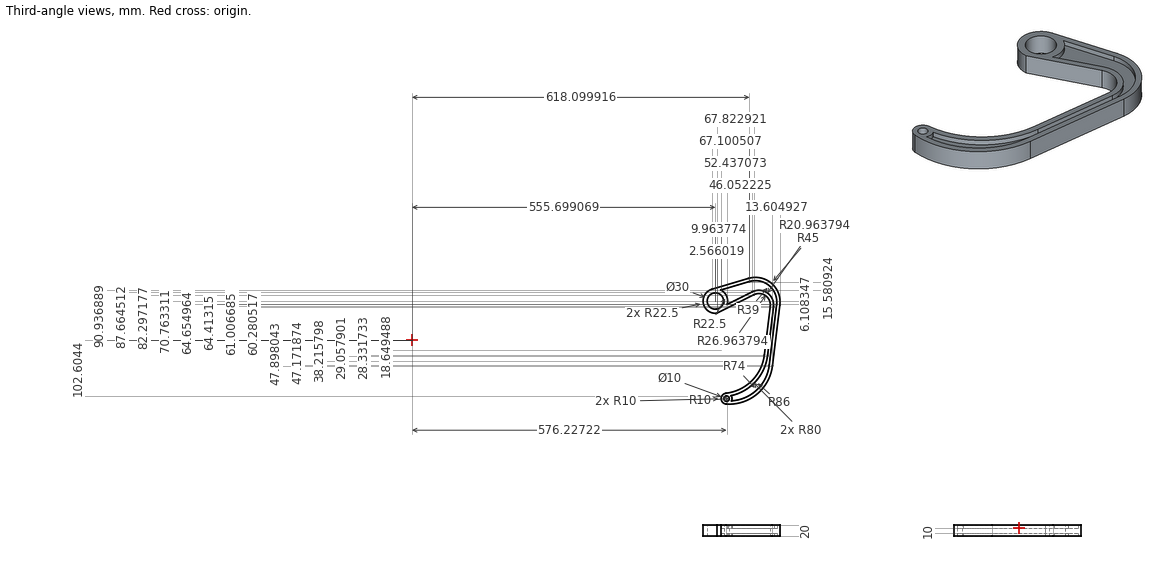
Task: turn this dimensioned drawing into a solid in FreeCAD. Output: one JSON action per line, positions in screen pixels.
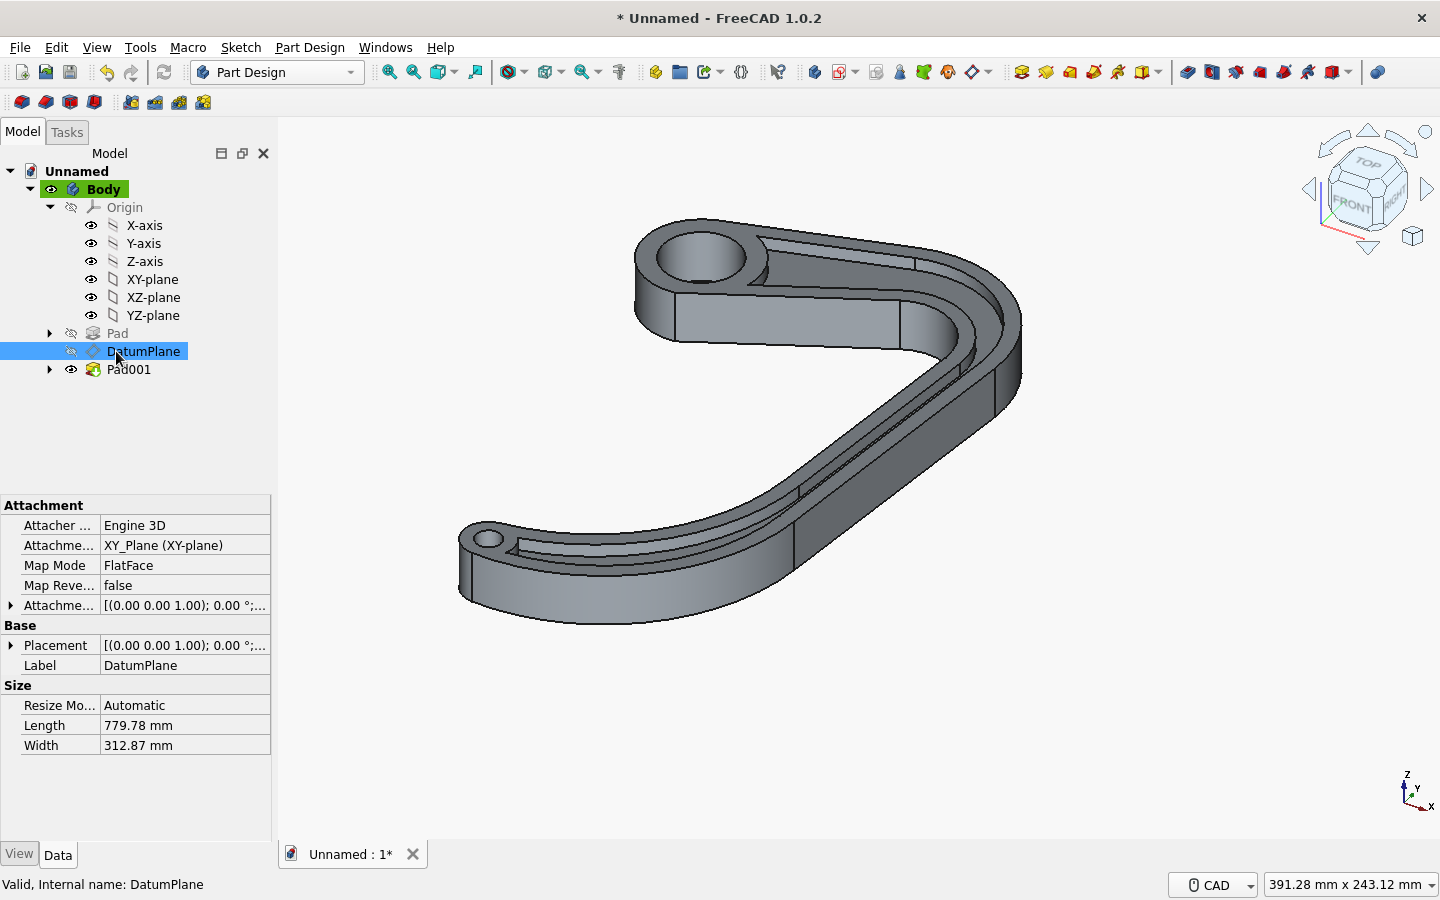
{"action": "key", "text": "0"}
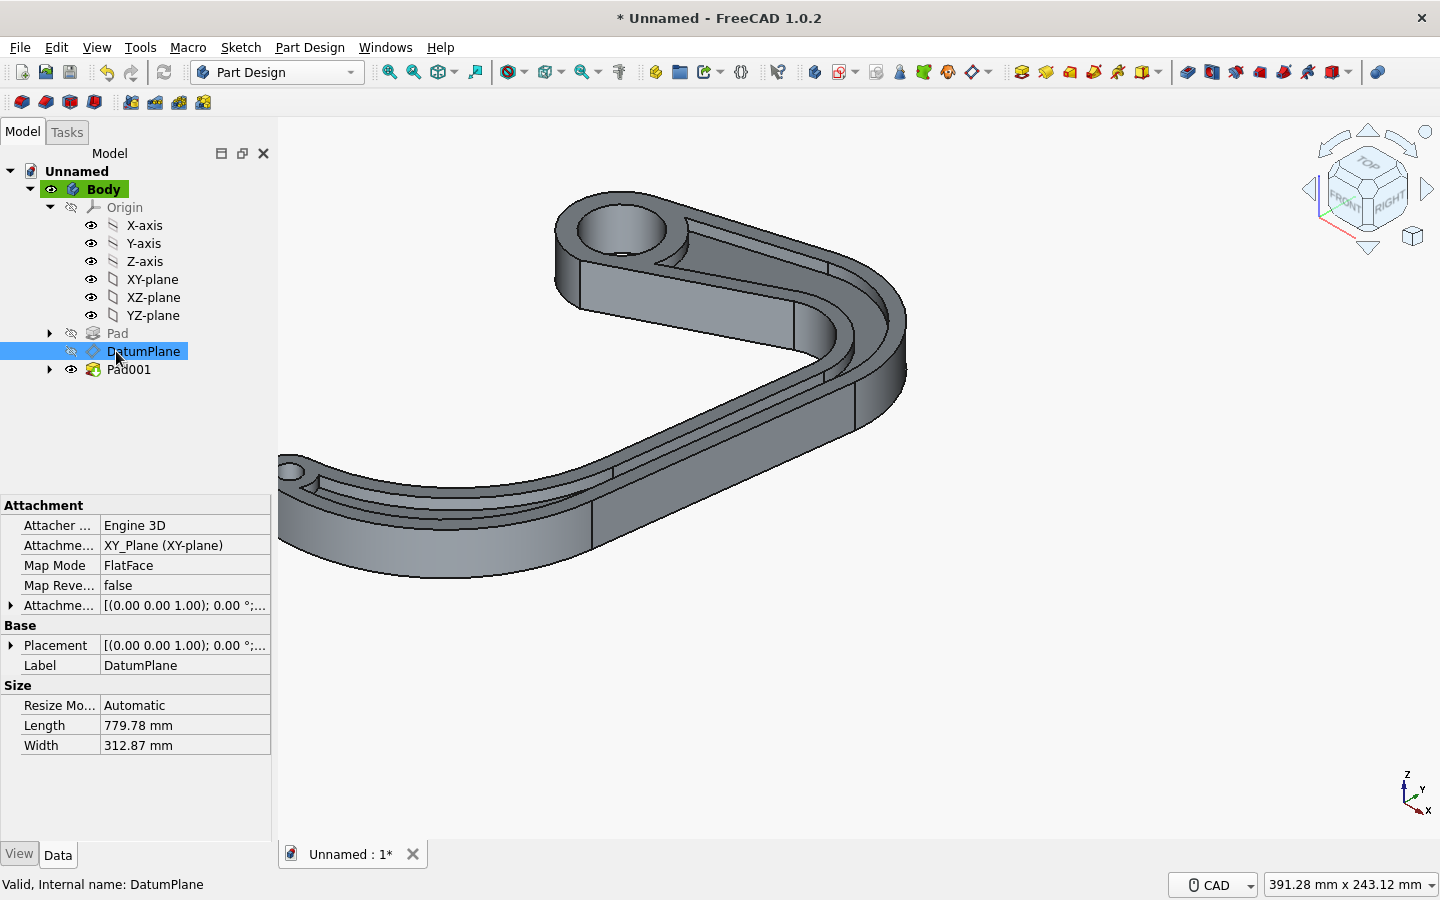
{"action": "left_click", "coordinate": [390, 72]}